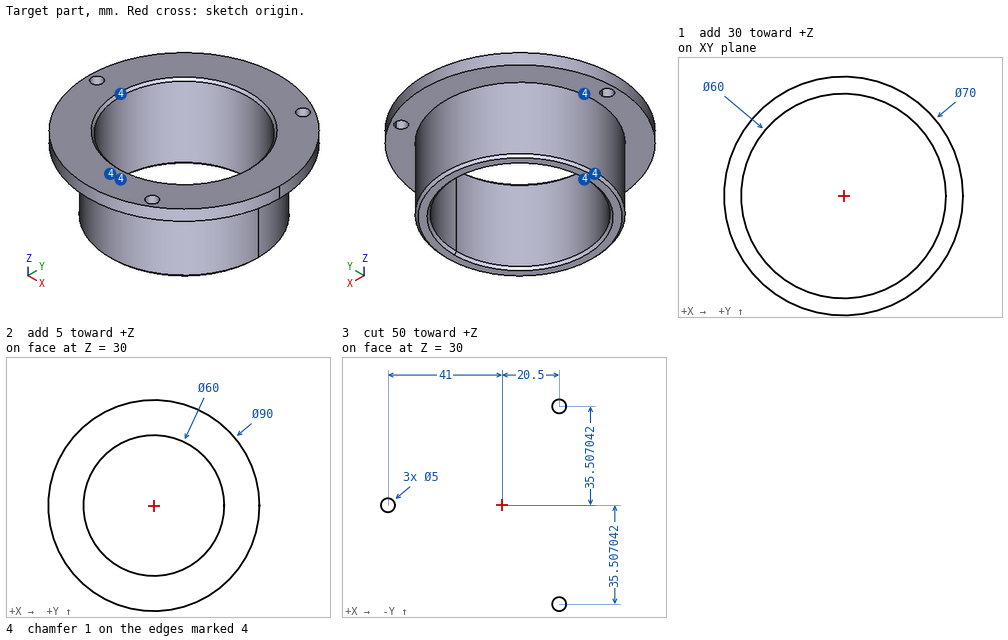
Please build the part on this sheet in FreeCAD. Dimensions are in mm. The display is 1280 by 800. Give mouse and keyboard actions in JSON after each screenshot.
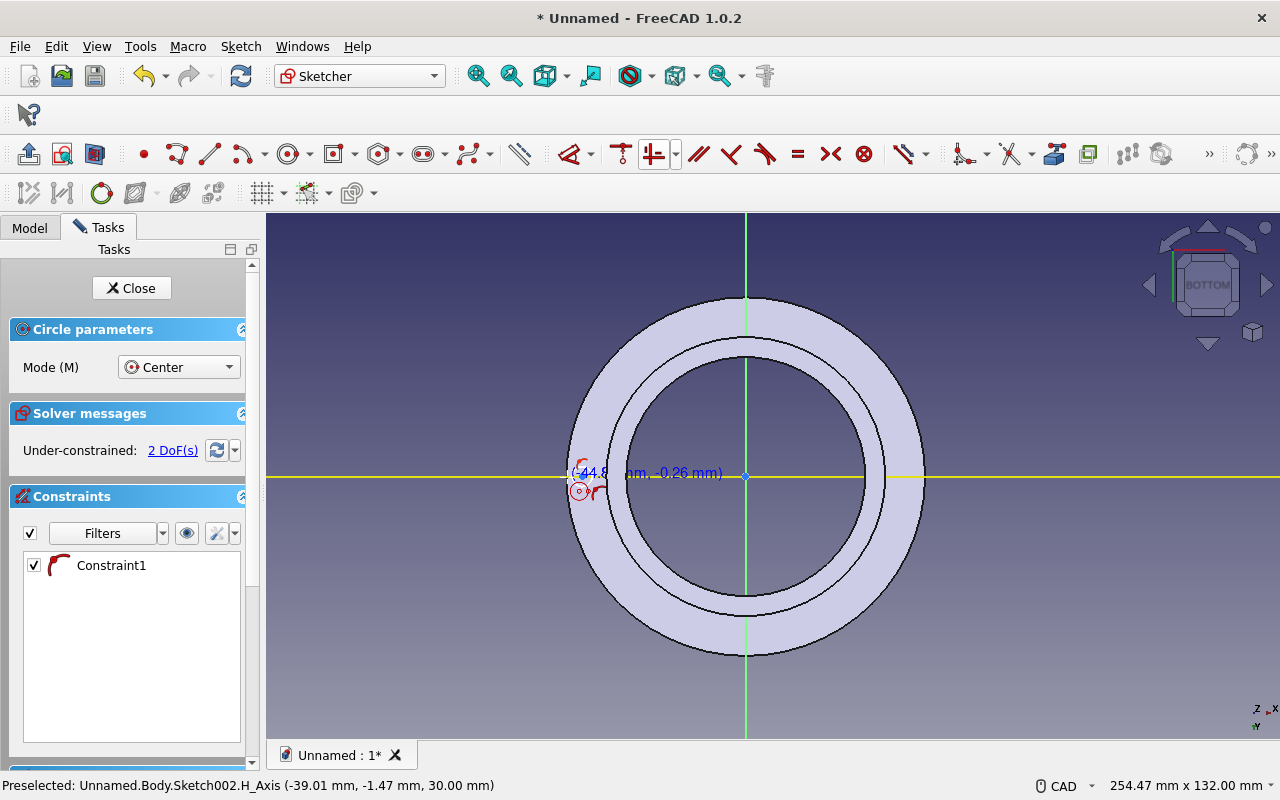
{"action": "scroll", "coordinate": [827, 335], "scroll_direction": "up", "scroll_amount": 5}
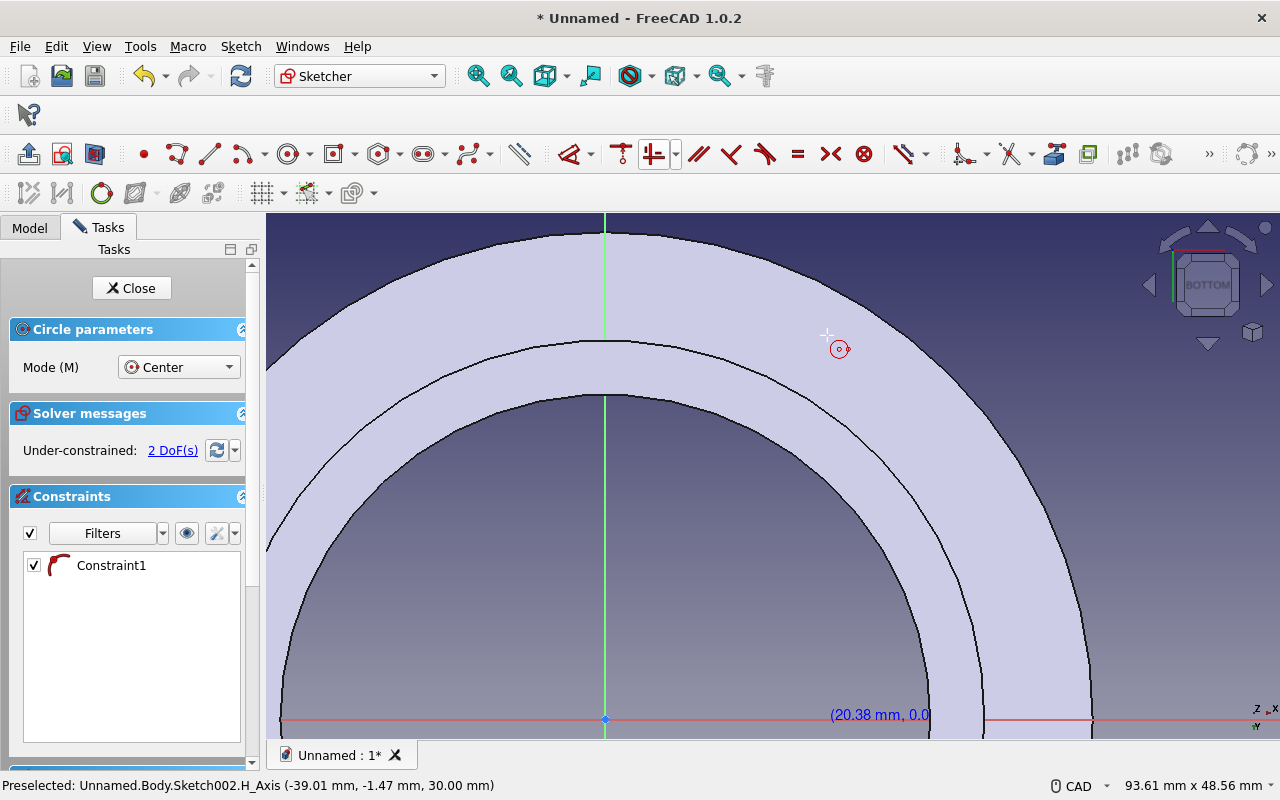
{"action": "left_click", "coordinate": [827, 335]}
{"action": "left_click", "coordinate": [846, 316]}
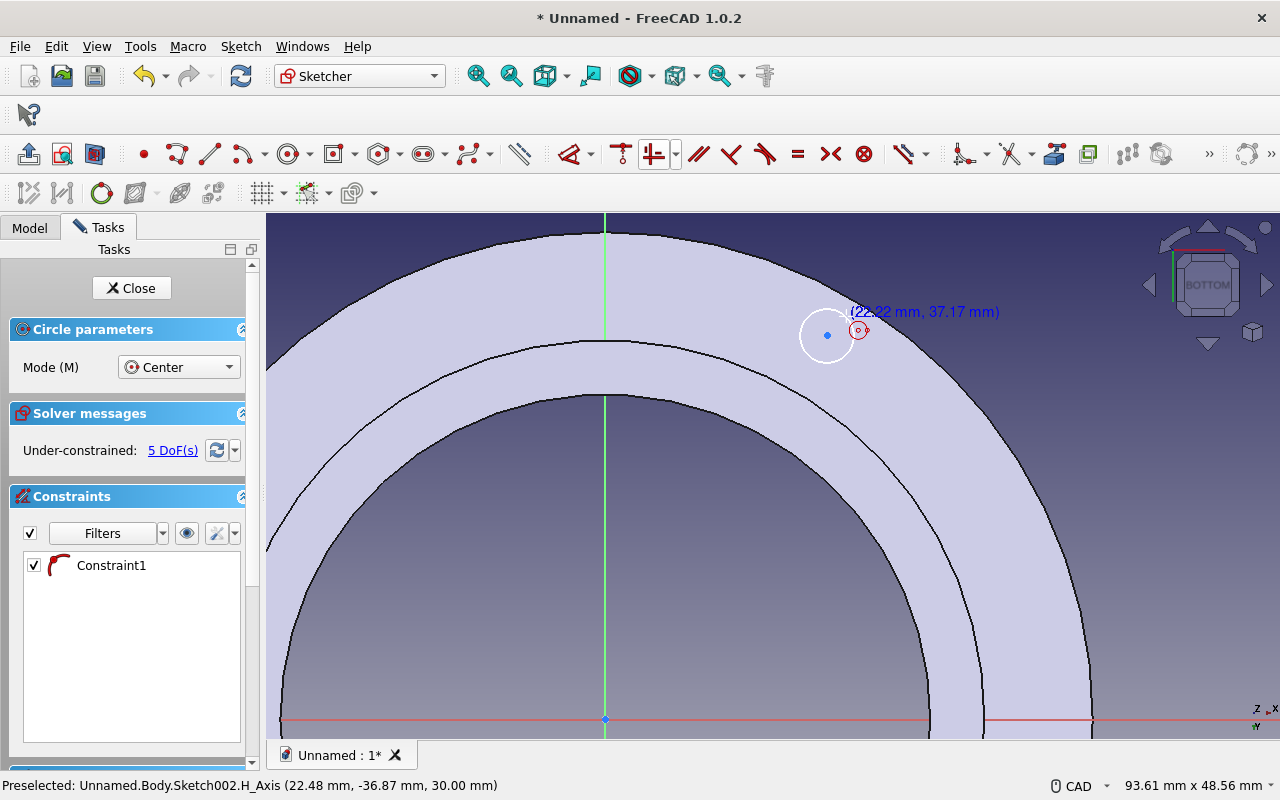
{"action": "scroll", "coordinate": [827, 334], "scroll_direction": "down", "scroll_amount": 5}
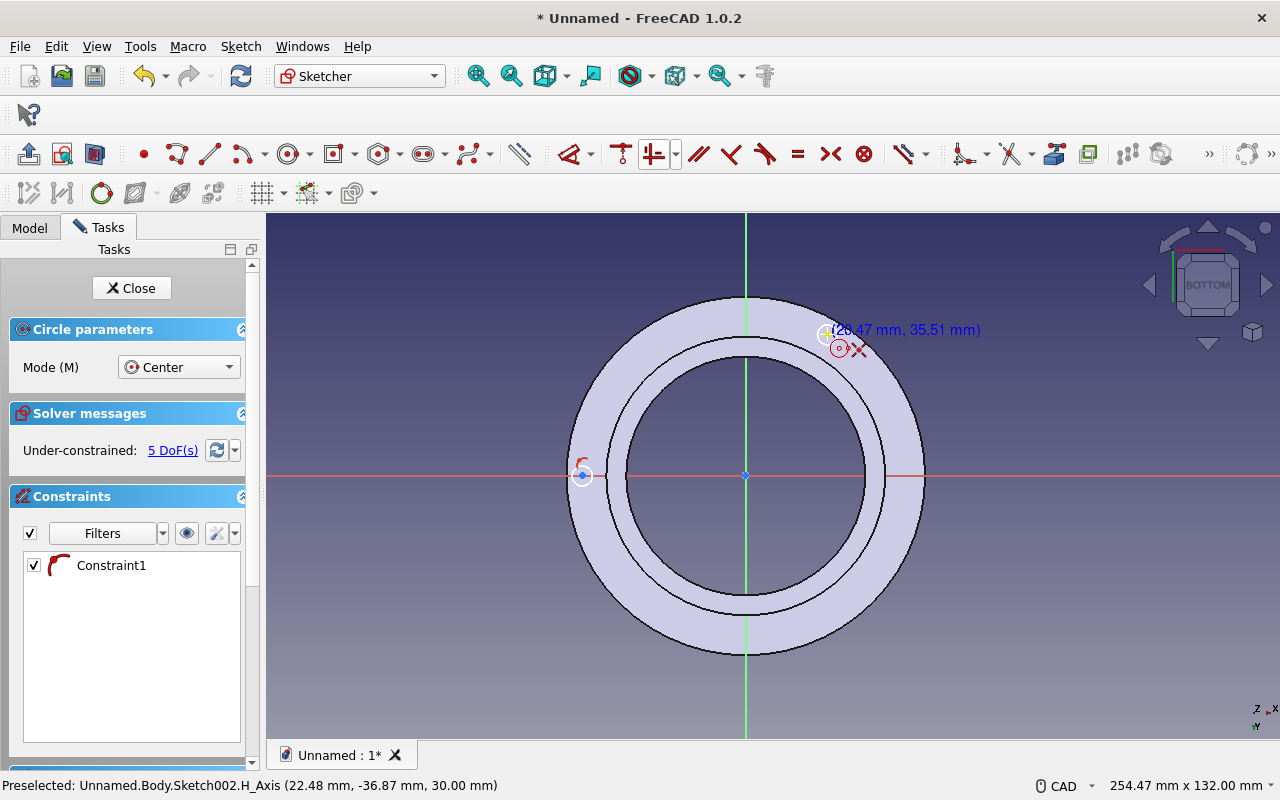
{"action": "scroll", "coordinate": [827, 617], "scroll_direction": "up", "scroll_amount": 5}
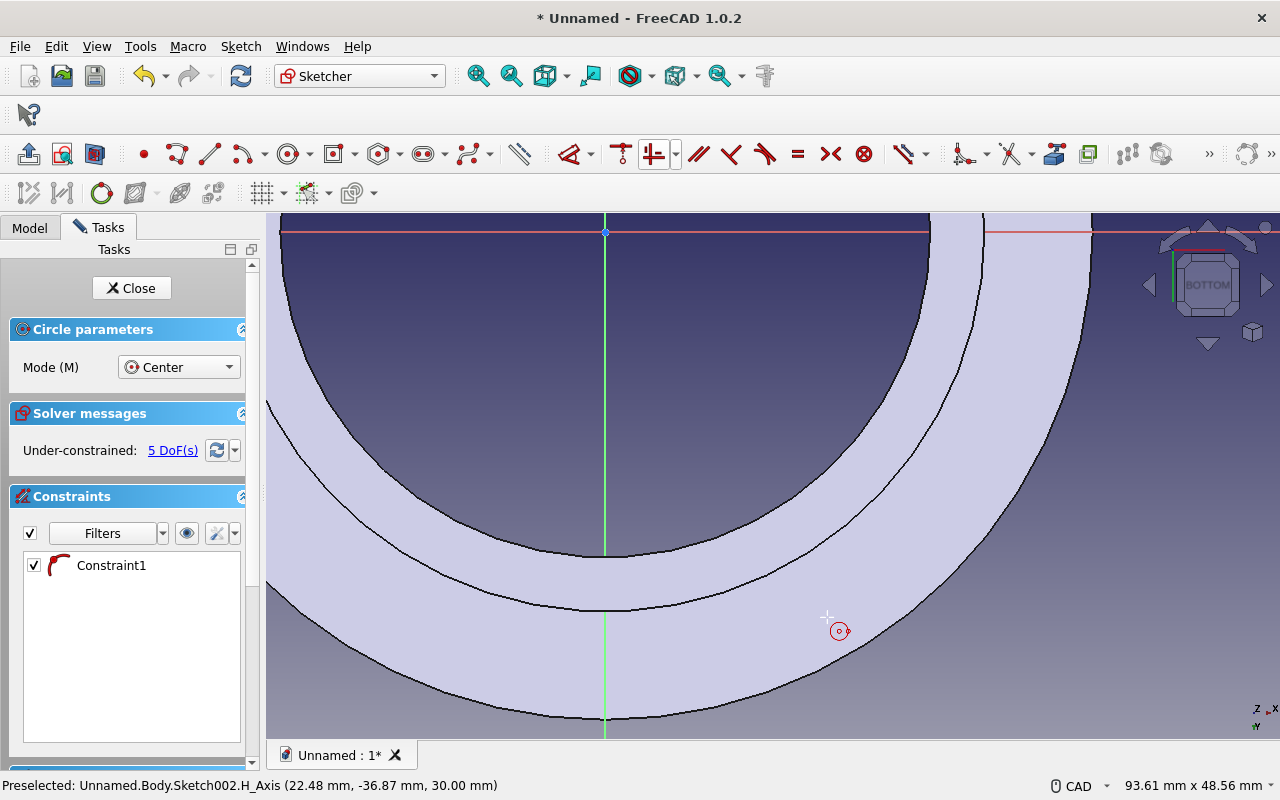
{"action": "left_click", "coordinate": [827, 617]}
{"action": "left_click", "coordinate": [846, 598]}
{"action": "key", "text": "Escape"}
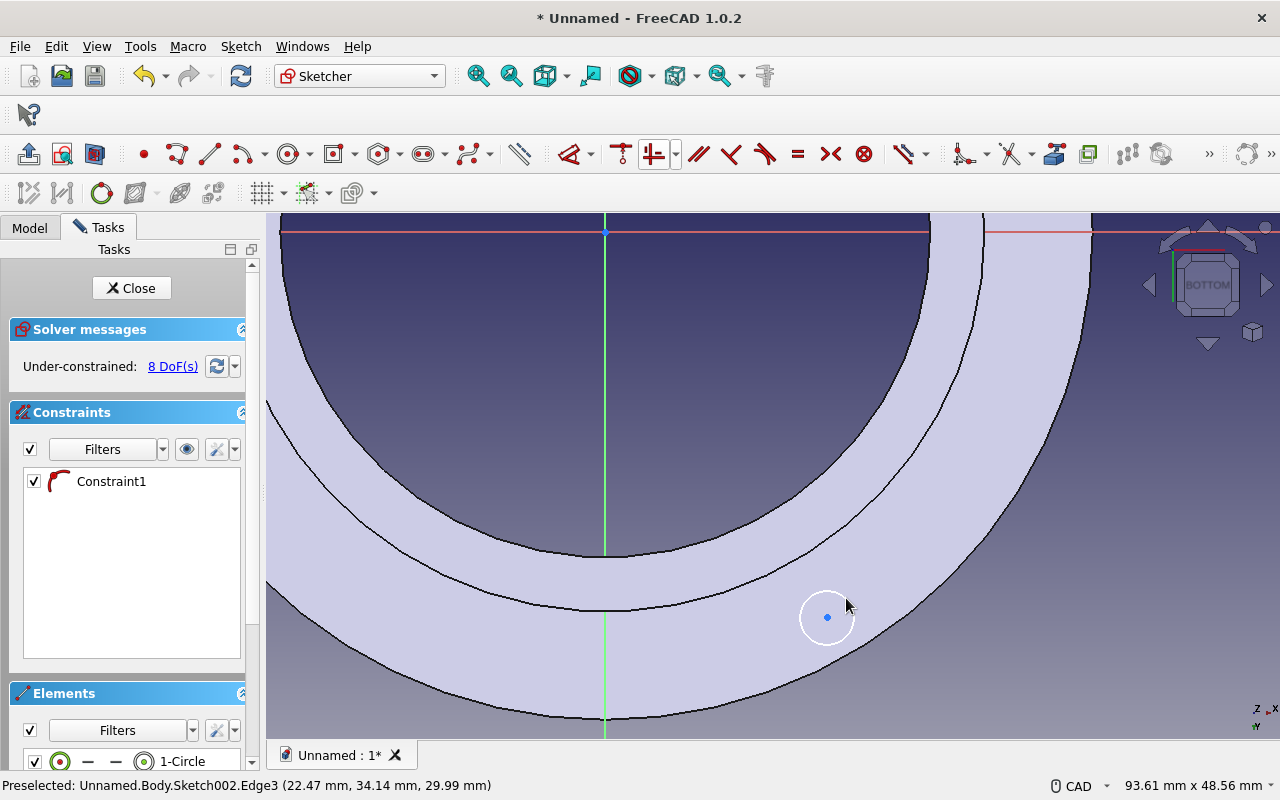
{"action": "scroll", "coordinate": [827, 618], "scroll_direction": "down", "scroll_amount": 5}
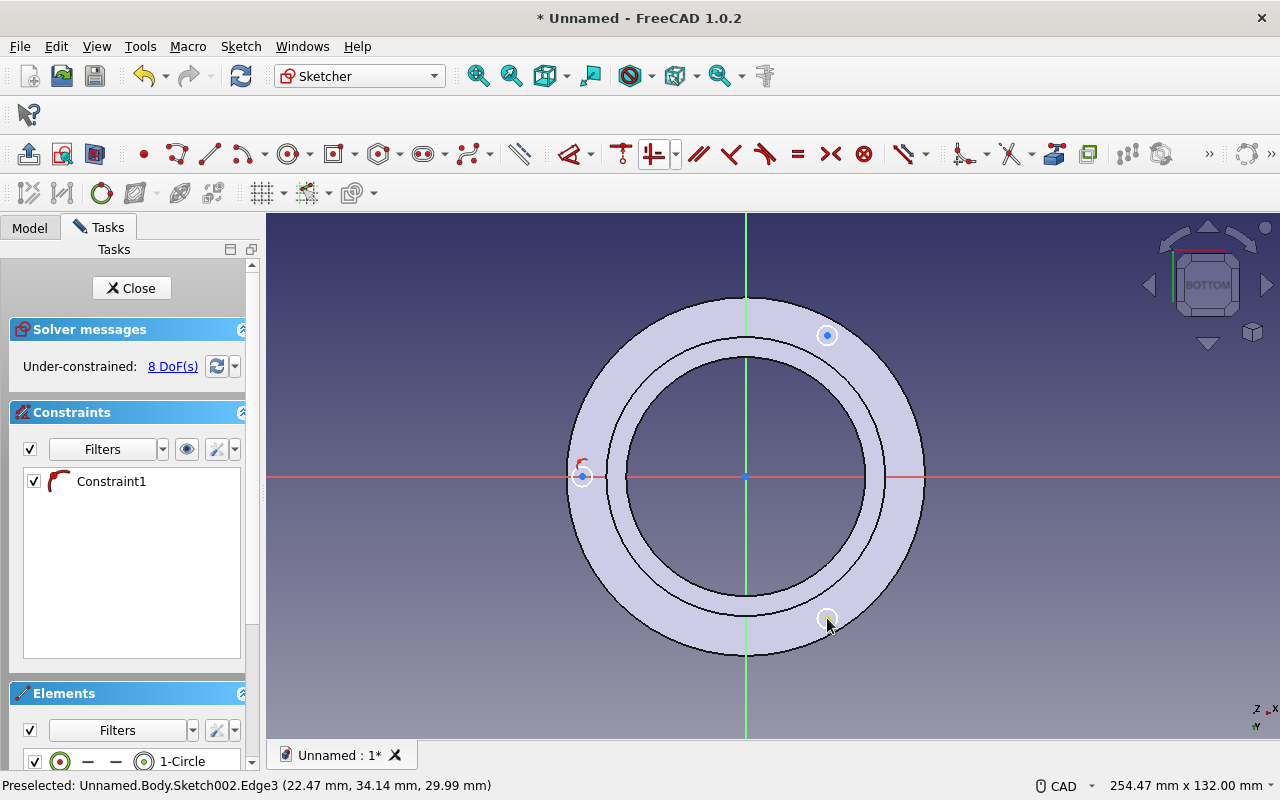
{"action": "scroll", "coordinate": [589, 470], "scroll_direction": "up", "scroll_amount": 4}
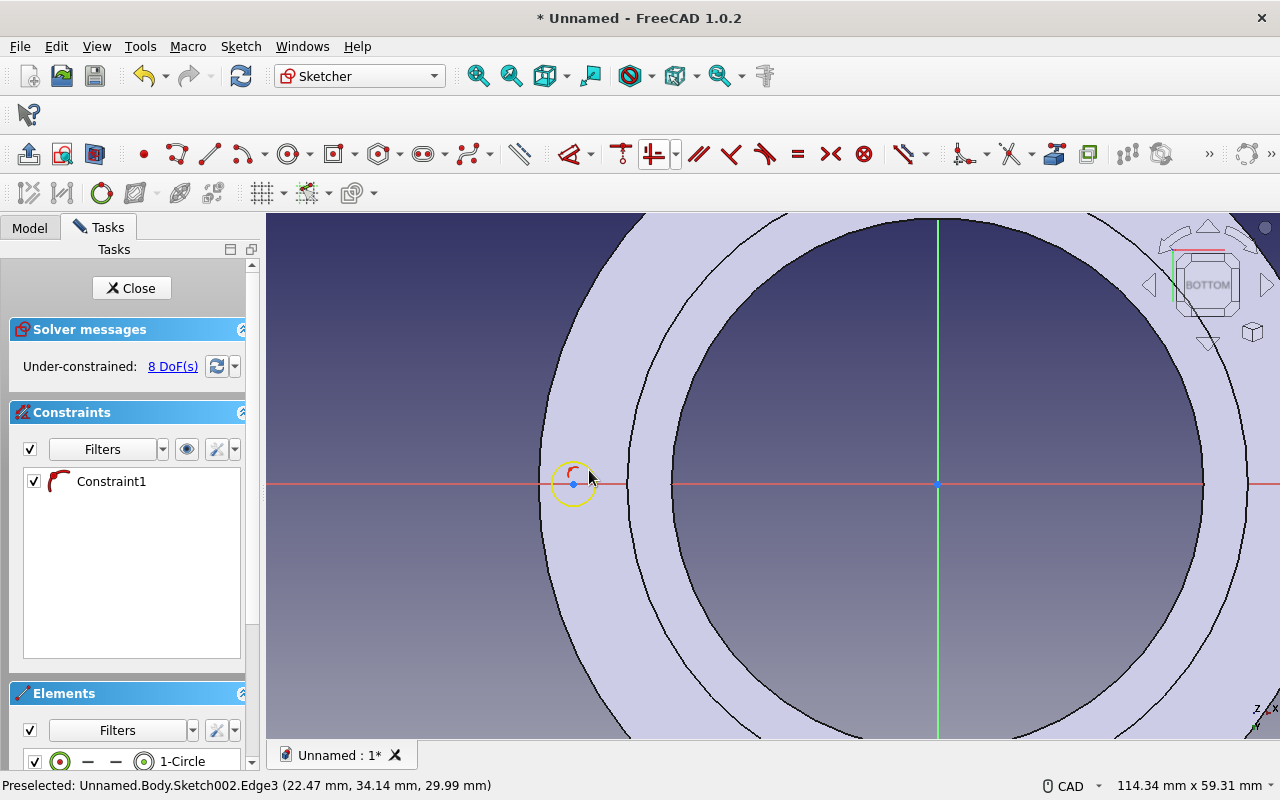
{"action": "left_click", "coordinate": [589, 468]}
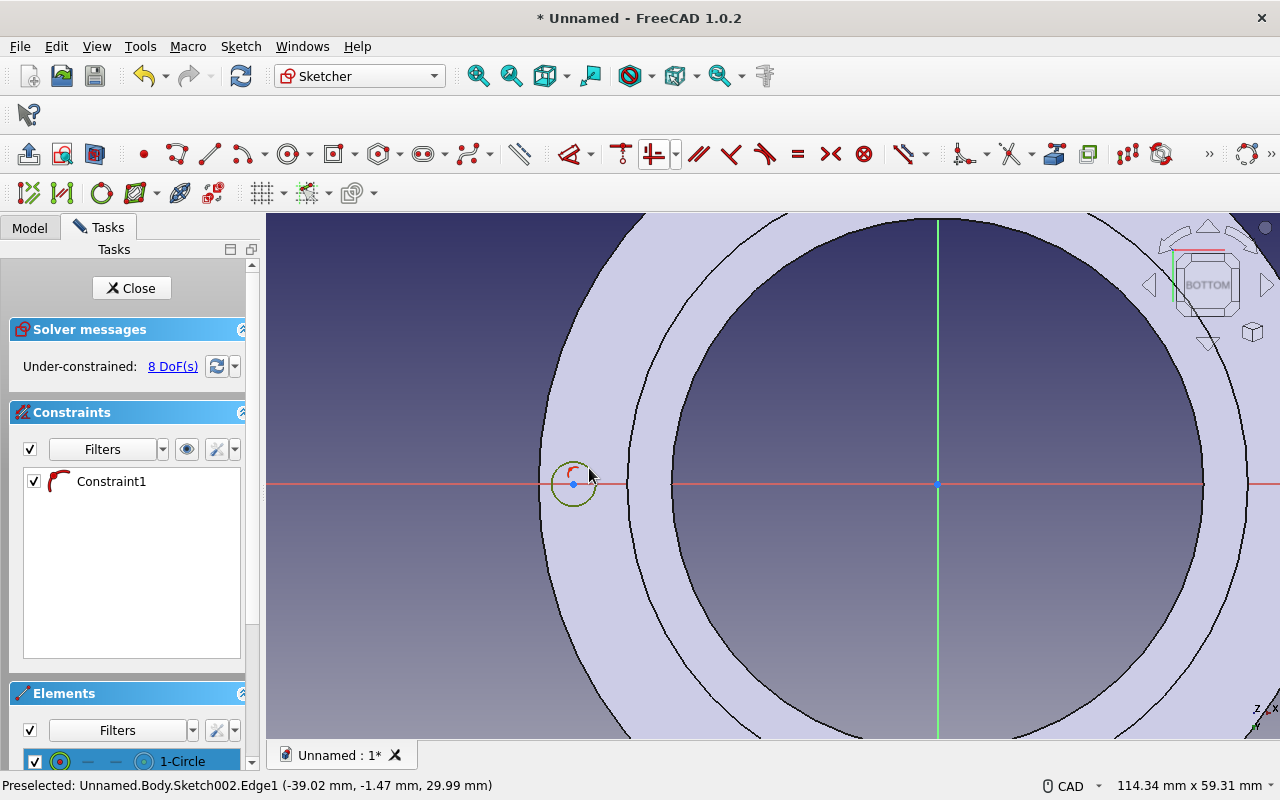
{"action": "scroll", "coordinate": [589, 469], "scroll_direction": "down", "scroll_amount": 4}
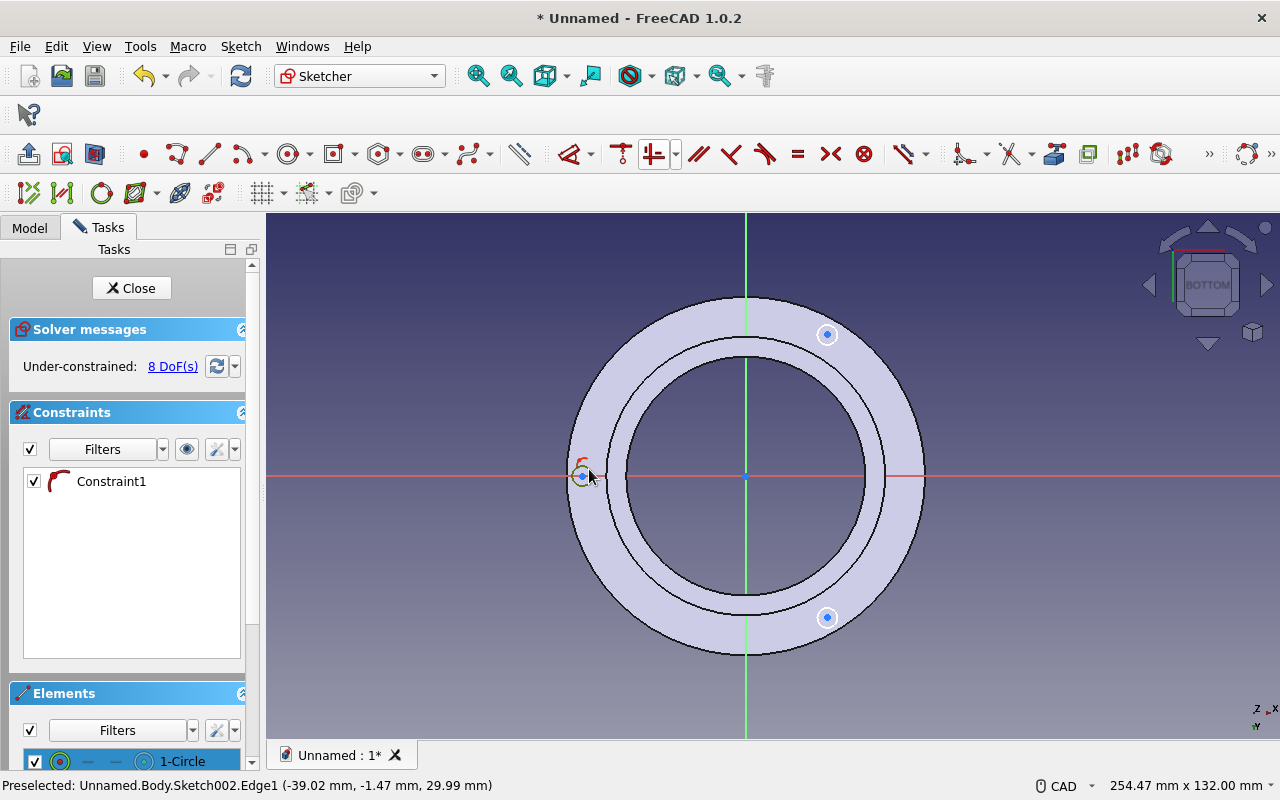
{"action": "scroll", "coordinate": [834, 328], "scroll_direction": "up", "scroll_amount": 2}